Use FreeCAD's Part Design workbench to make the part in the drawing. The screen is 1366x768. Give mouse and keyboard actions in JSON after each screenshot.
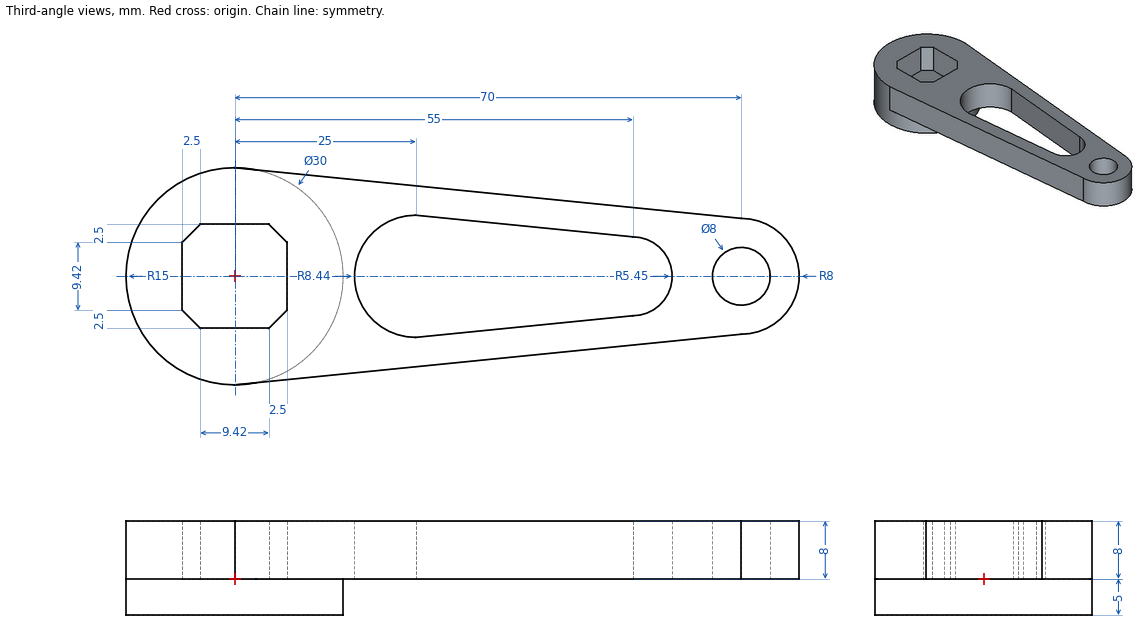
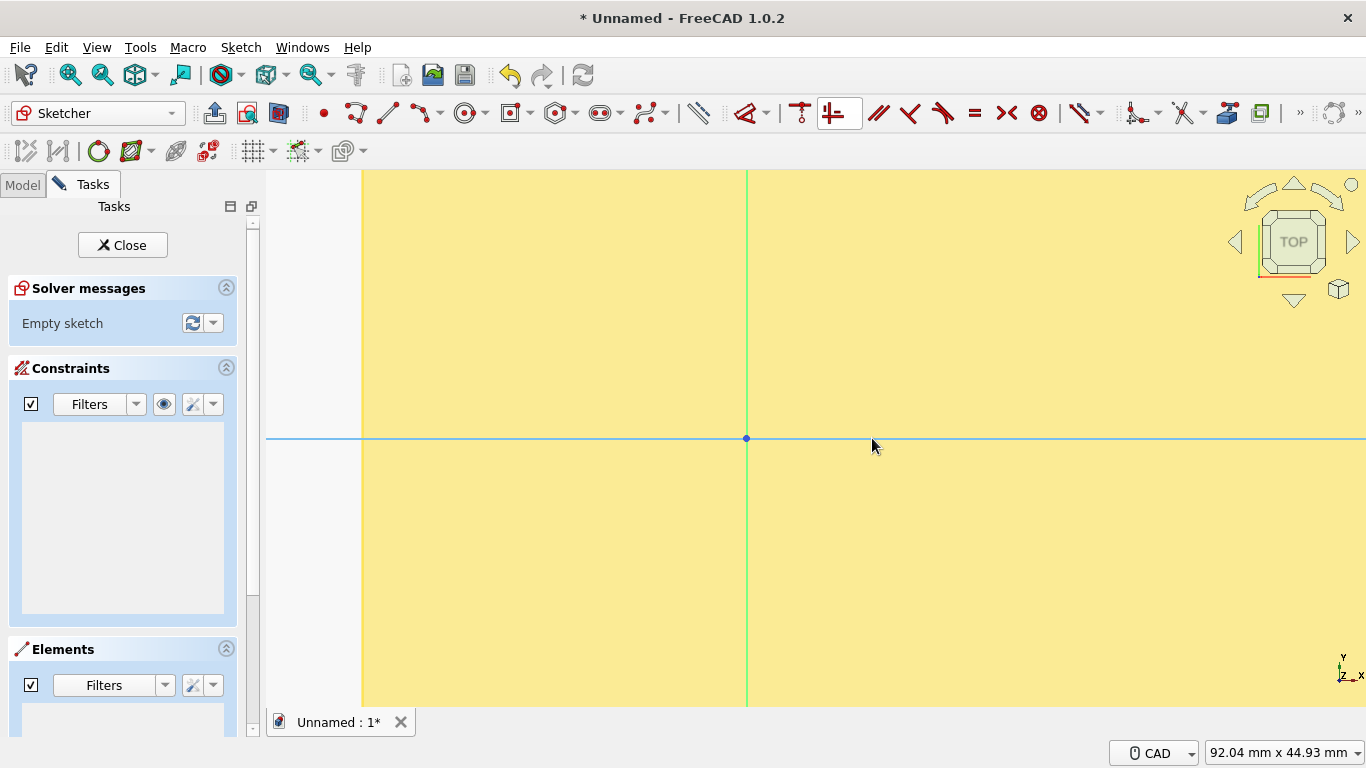
{"action": "left_click", "coordinate": [466, 114]}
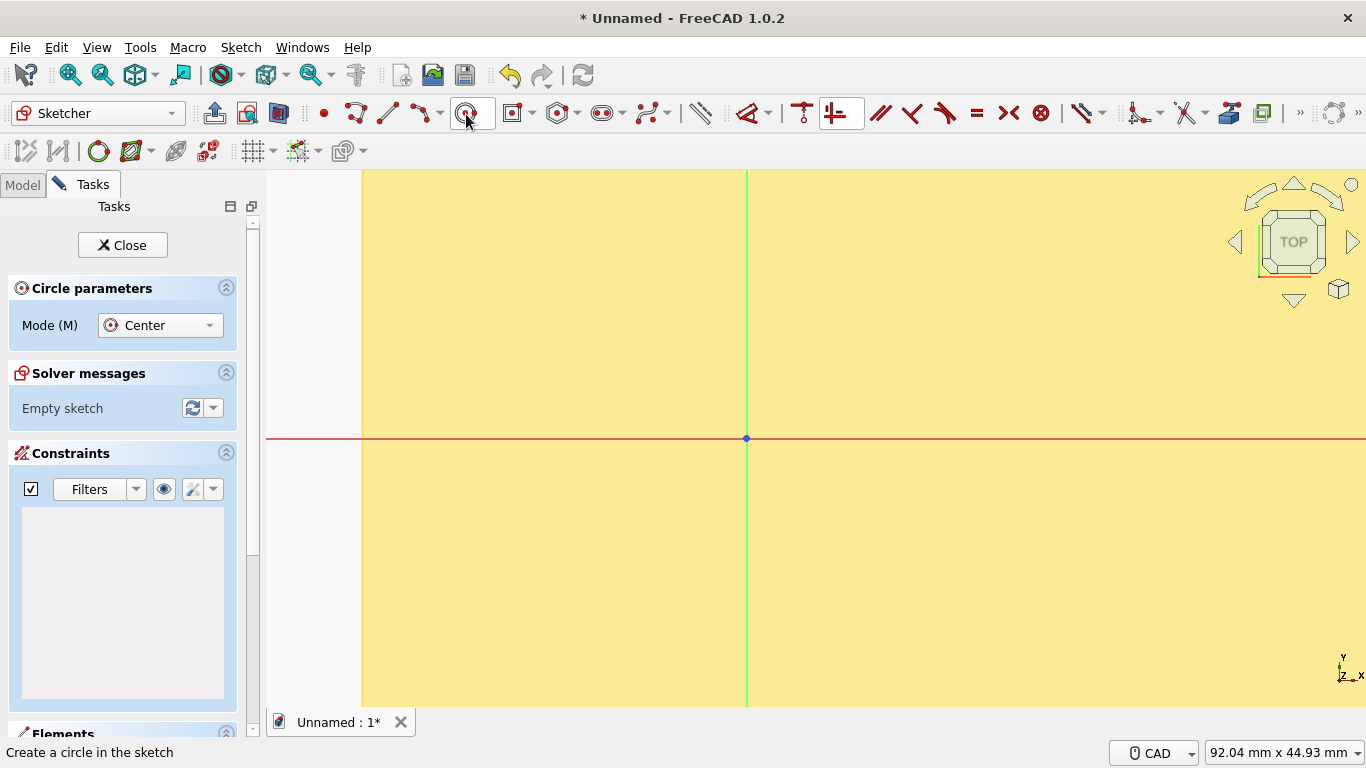
{"action": "left_click", "coordinate": [747, 438]}
{"action": "left_click", "coordinate": [873, 312]}
{"action": "key", "text": "Escape"}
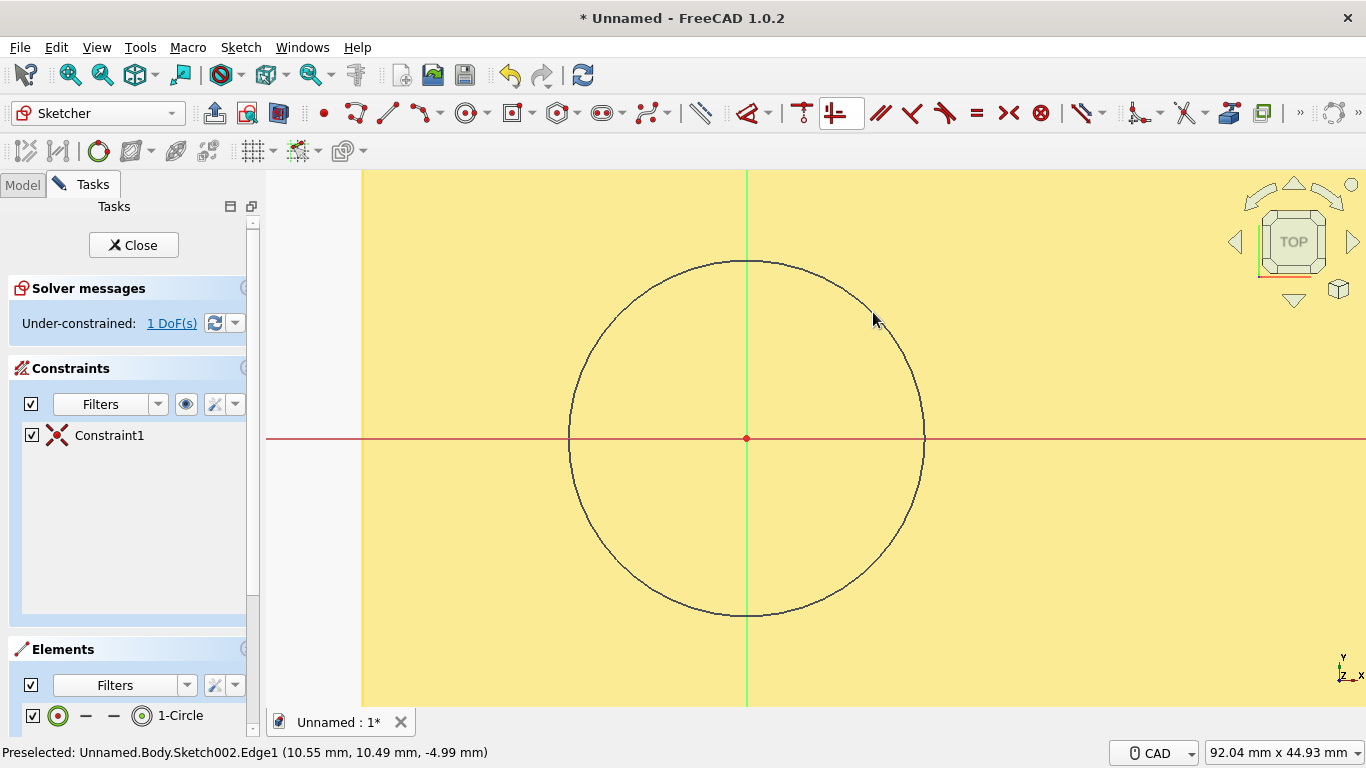
{"action": "left_click", "coordinate": [748, 114]}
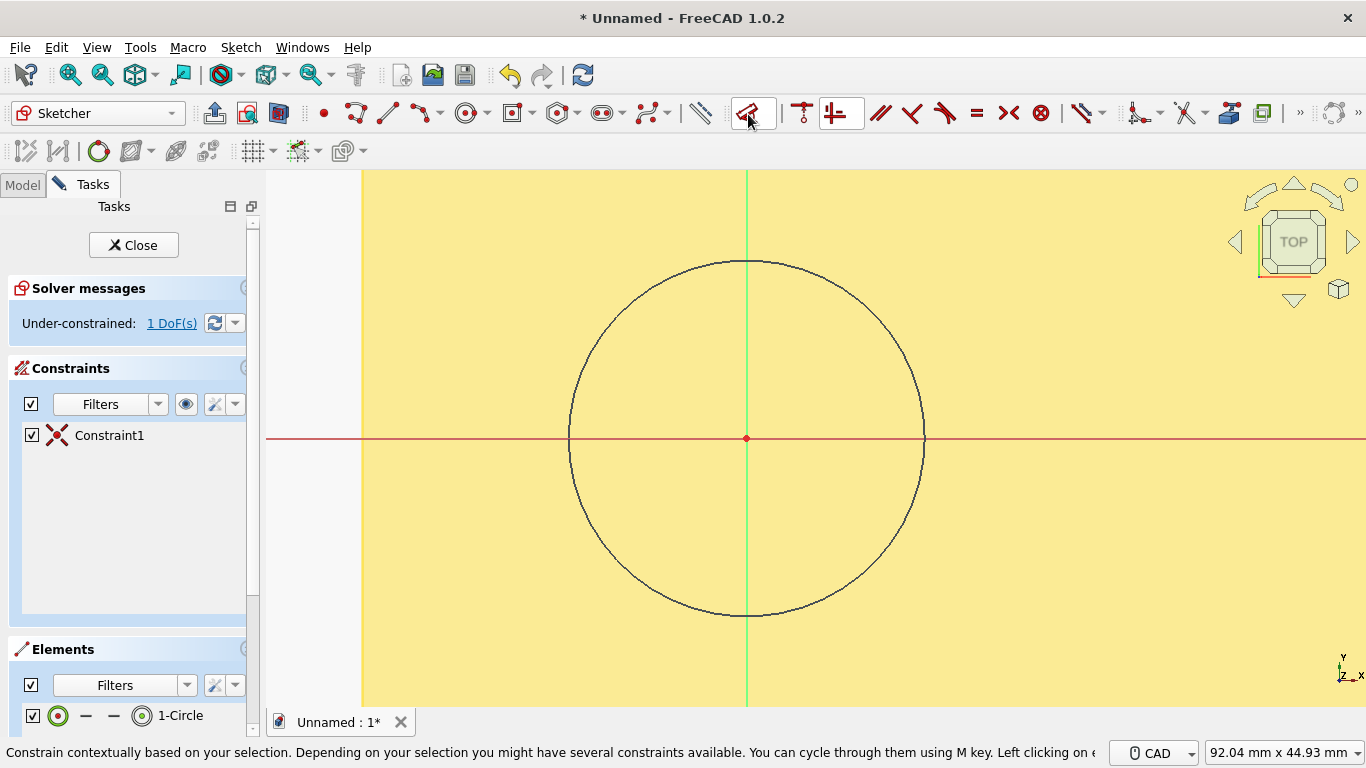
{"action": "left_click", "coordinate": [872, 312]}
{"action": "left_click", "coordinate": [895, 289]}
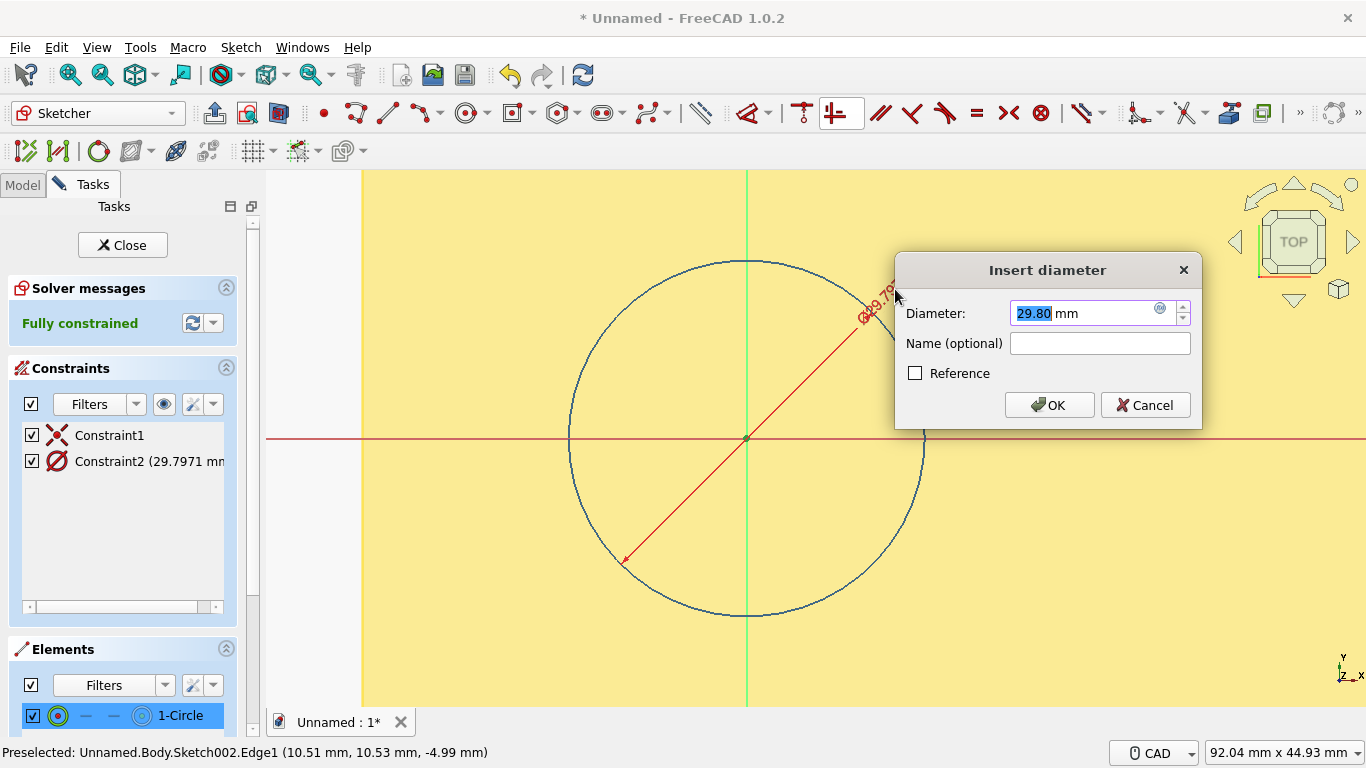
{"action": "type", "text": "30"}
{"action": "key", "text": "Return"}
{"action": "key", "text": "Escape"}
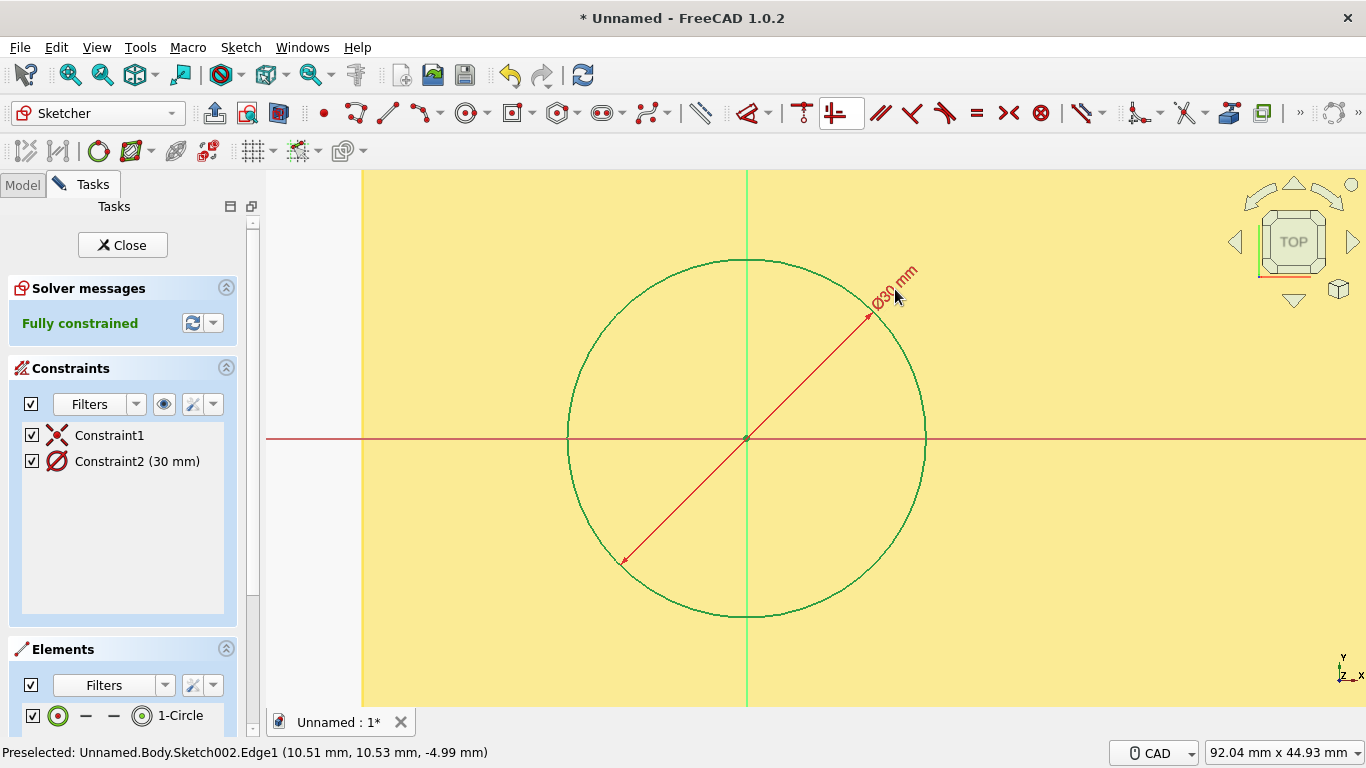
{"action": "left_click", "coordinate": [123, 245]}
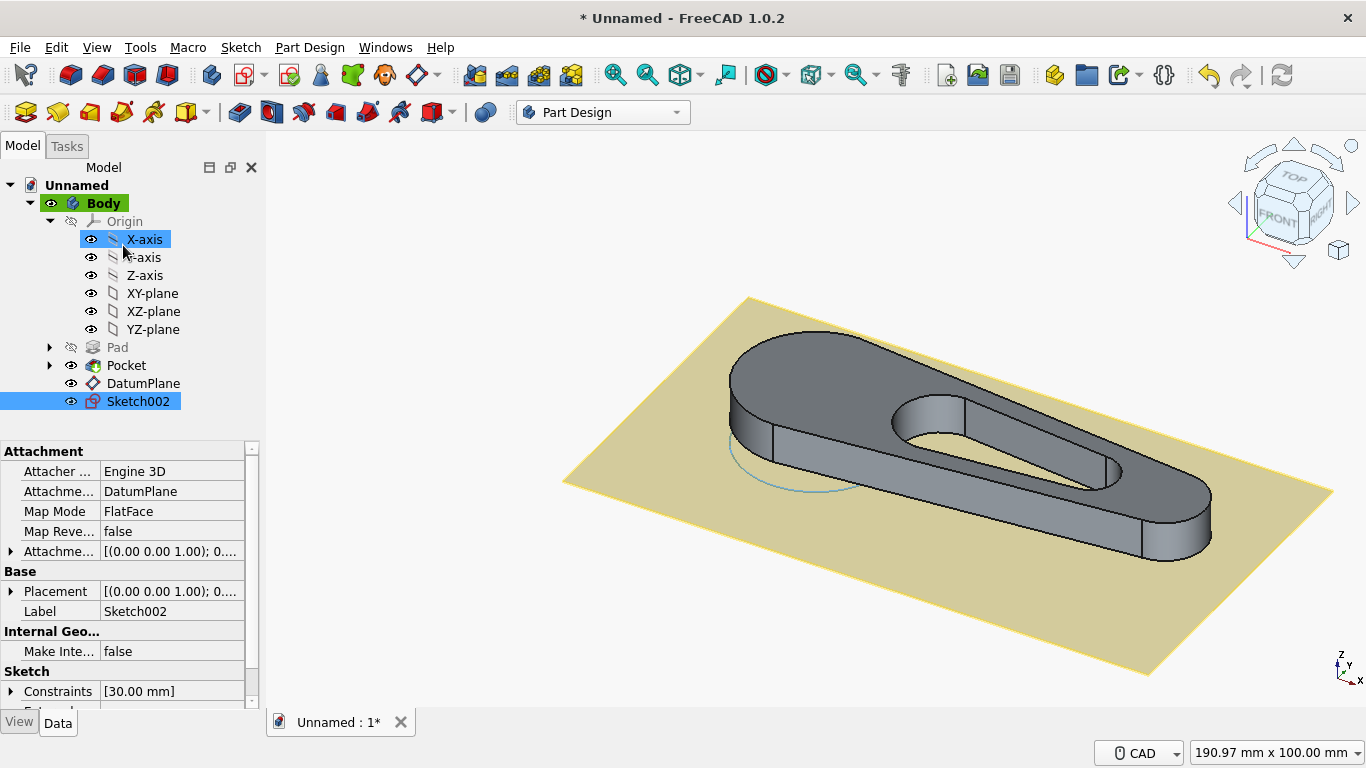
{"action": "left_click", "coordinate": [26, 112]}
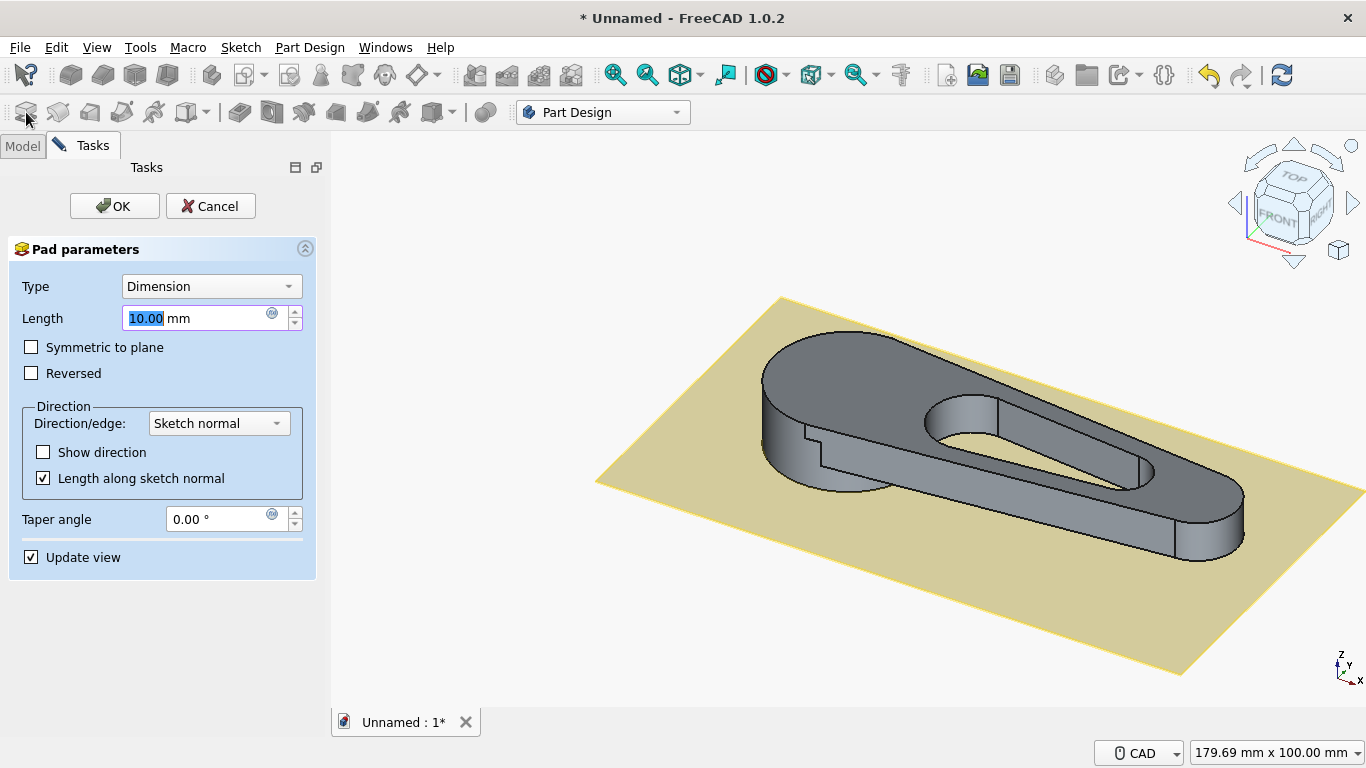
{"action": "type", "text": "5"}
{"action": "key", "text": "Tab"}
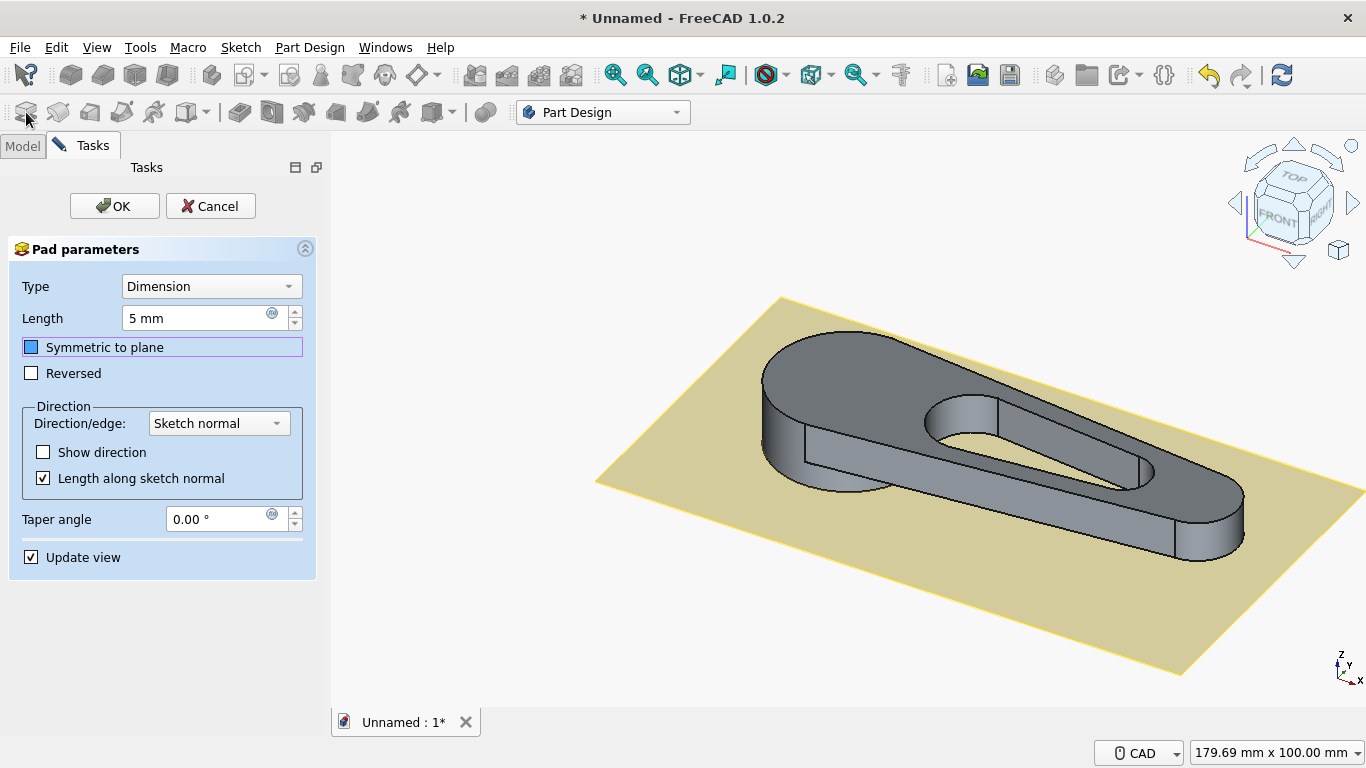
{"action": "left_click", "coordinate": [115, 206]}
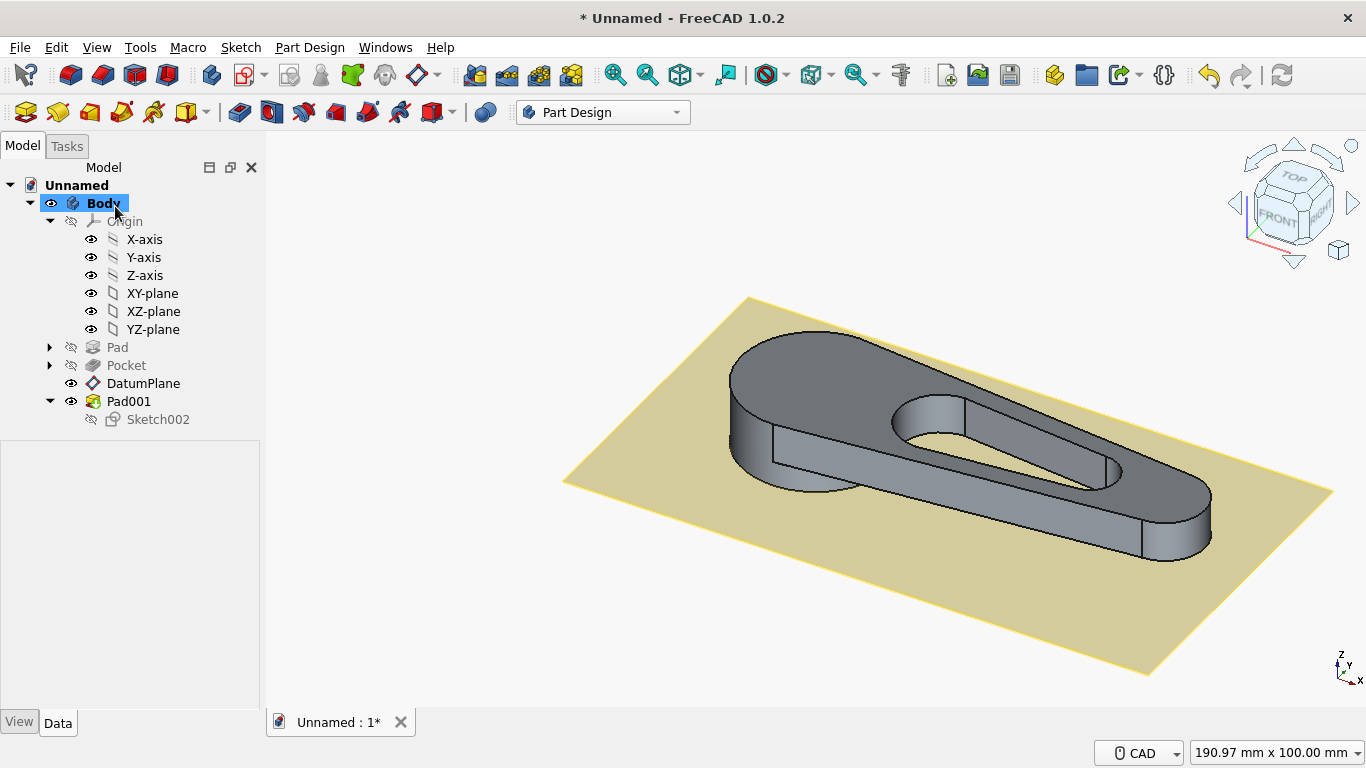
{"action": "left_click", "coordinate": [116, 383]}
{"action": "key", "text": "space"}